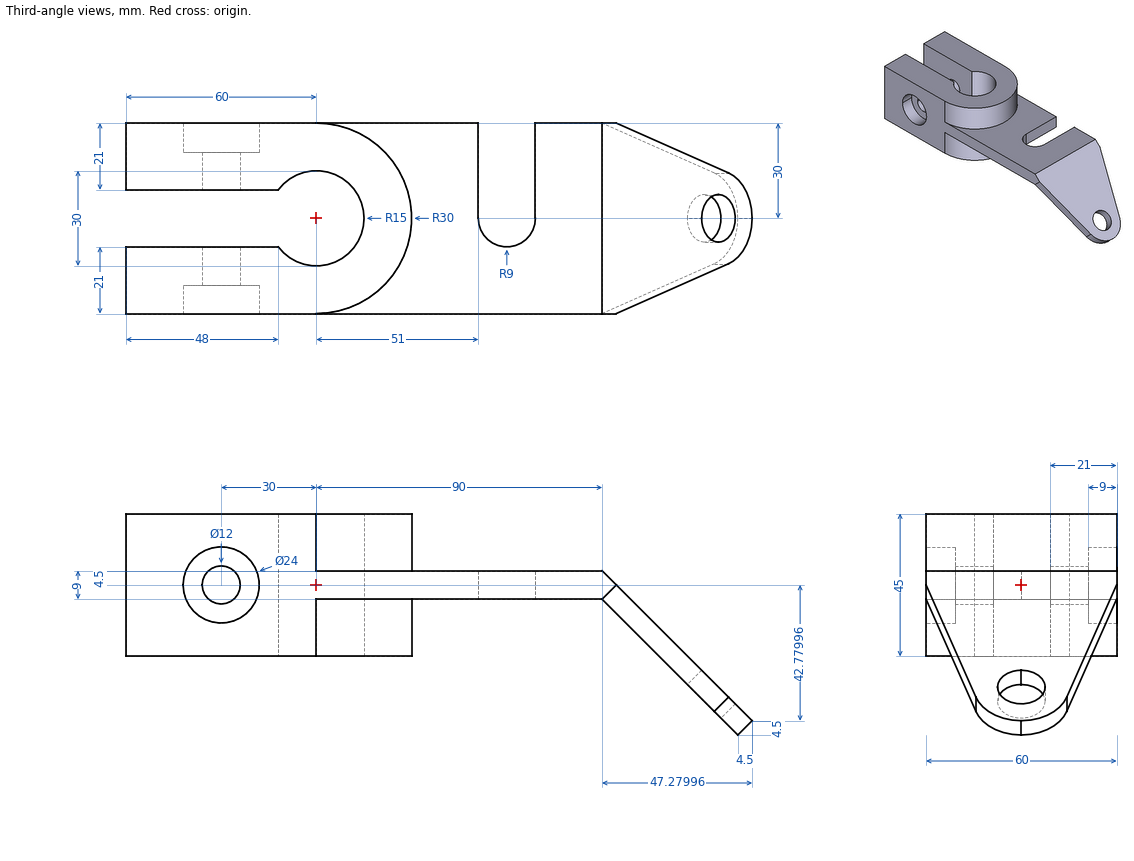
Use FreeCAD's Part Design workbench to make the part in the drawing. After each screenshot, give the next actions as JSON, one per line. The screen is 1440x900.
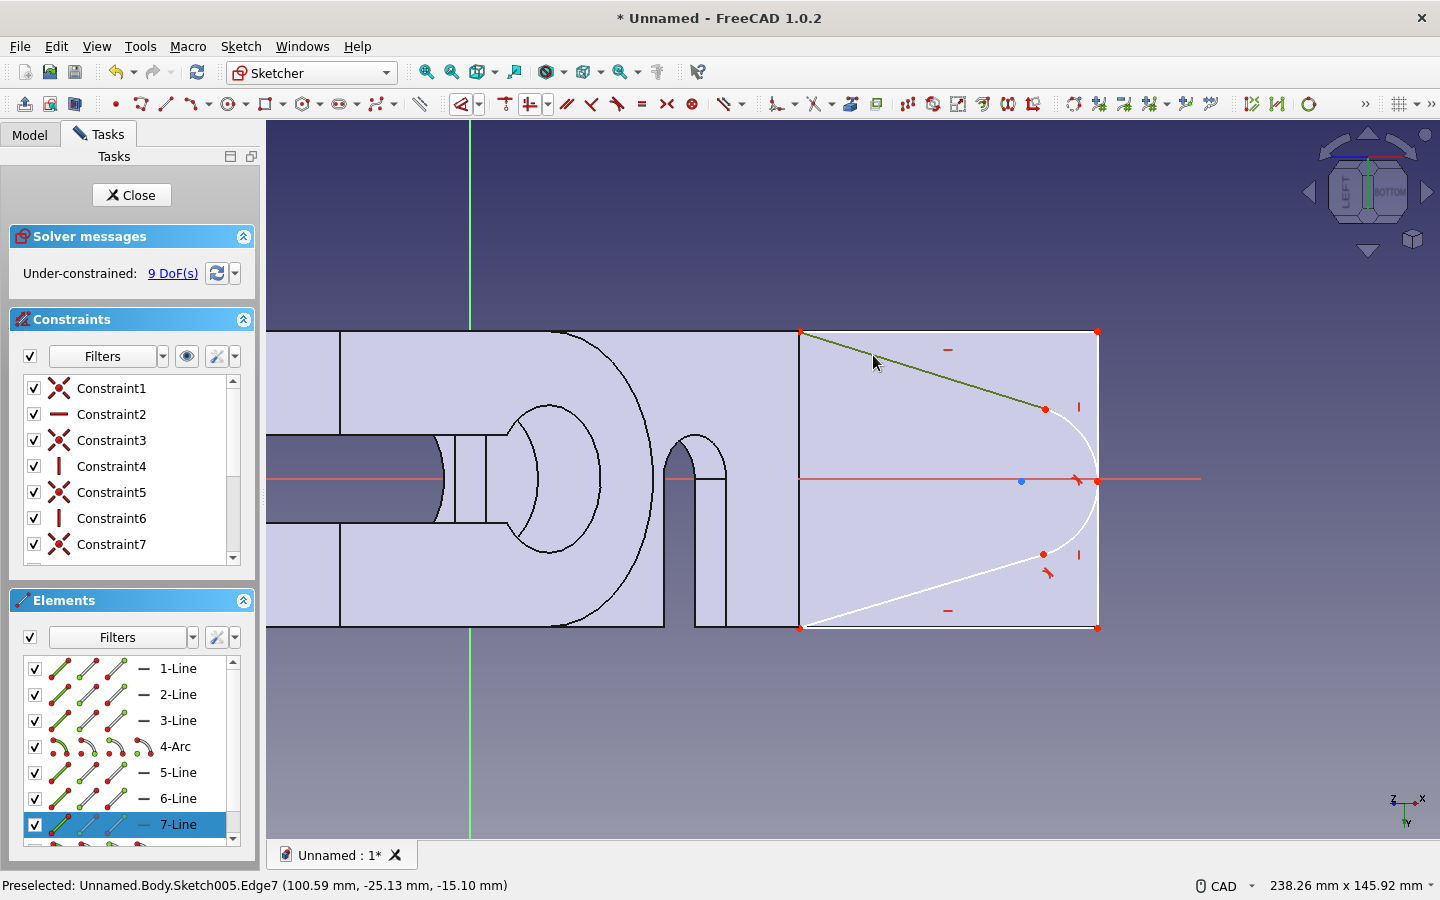
{"action": "left_click", "coordinate": [1071, 423]}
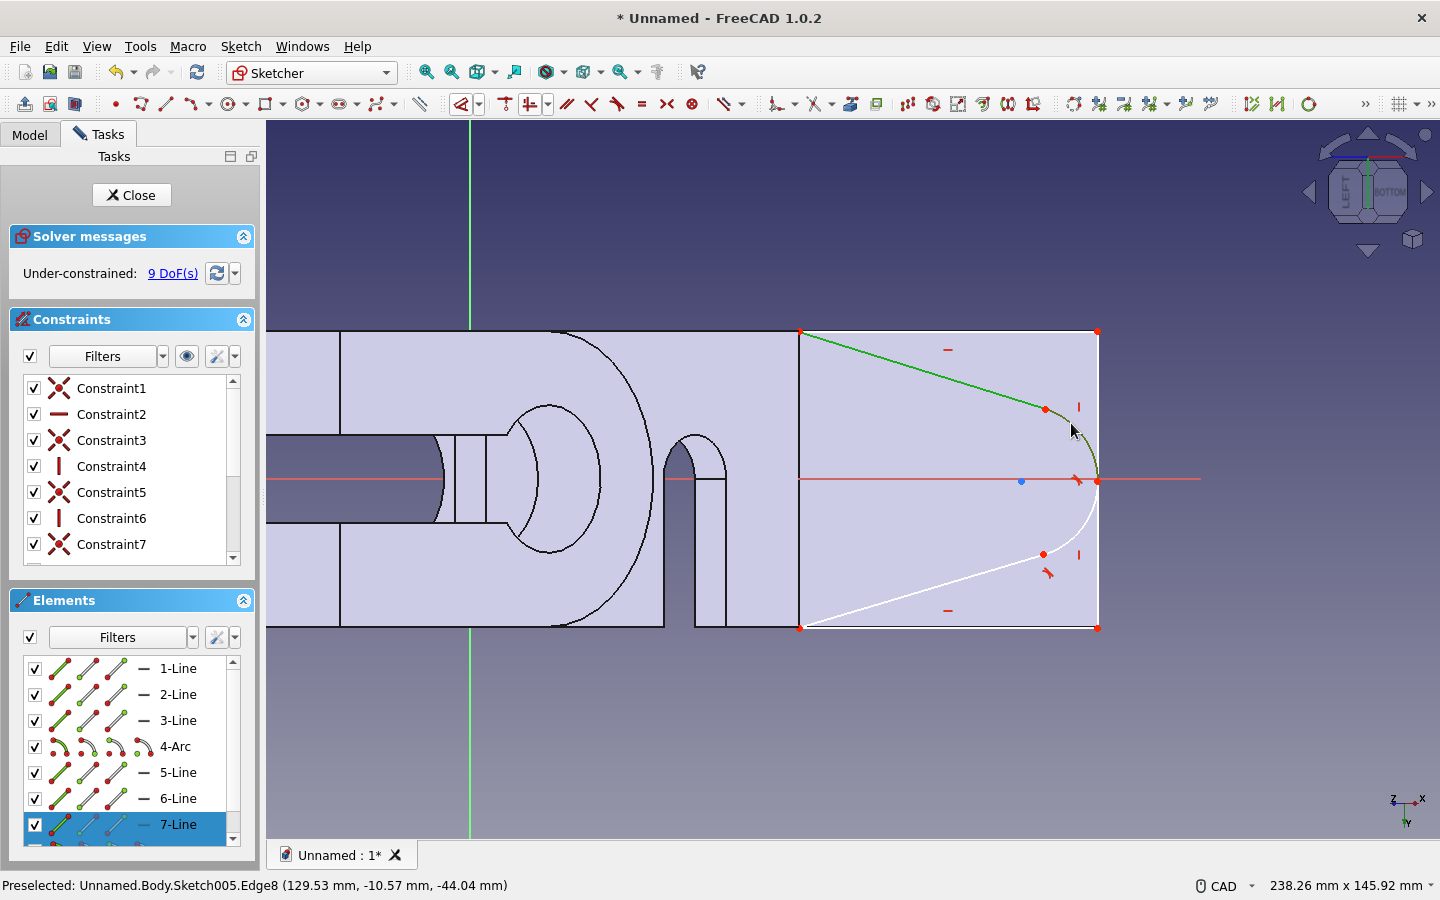
{"action": "left_click", "coordinate": [617, 104]}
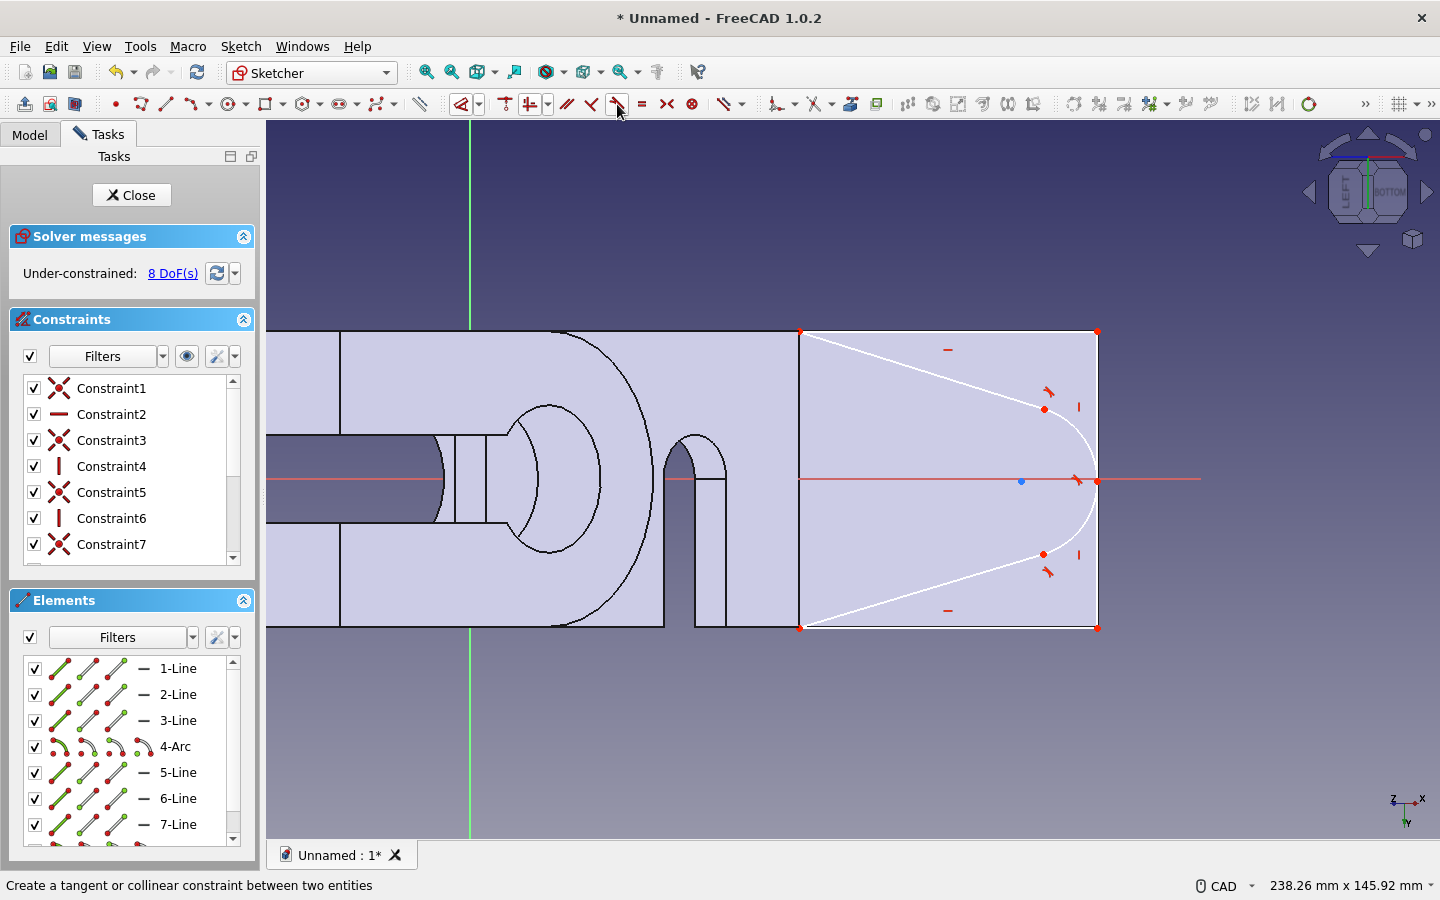
{"action": "left_click", "coordinate": [1069, 541]}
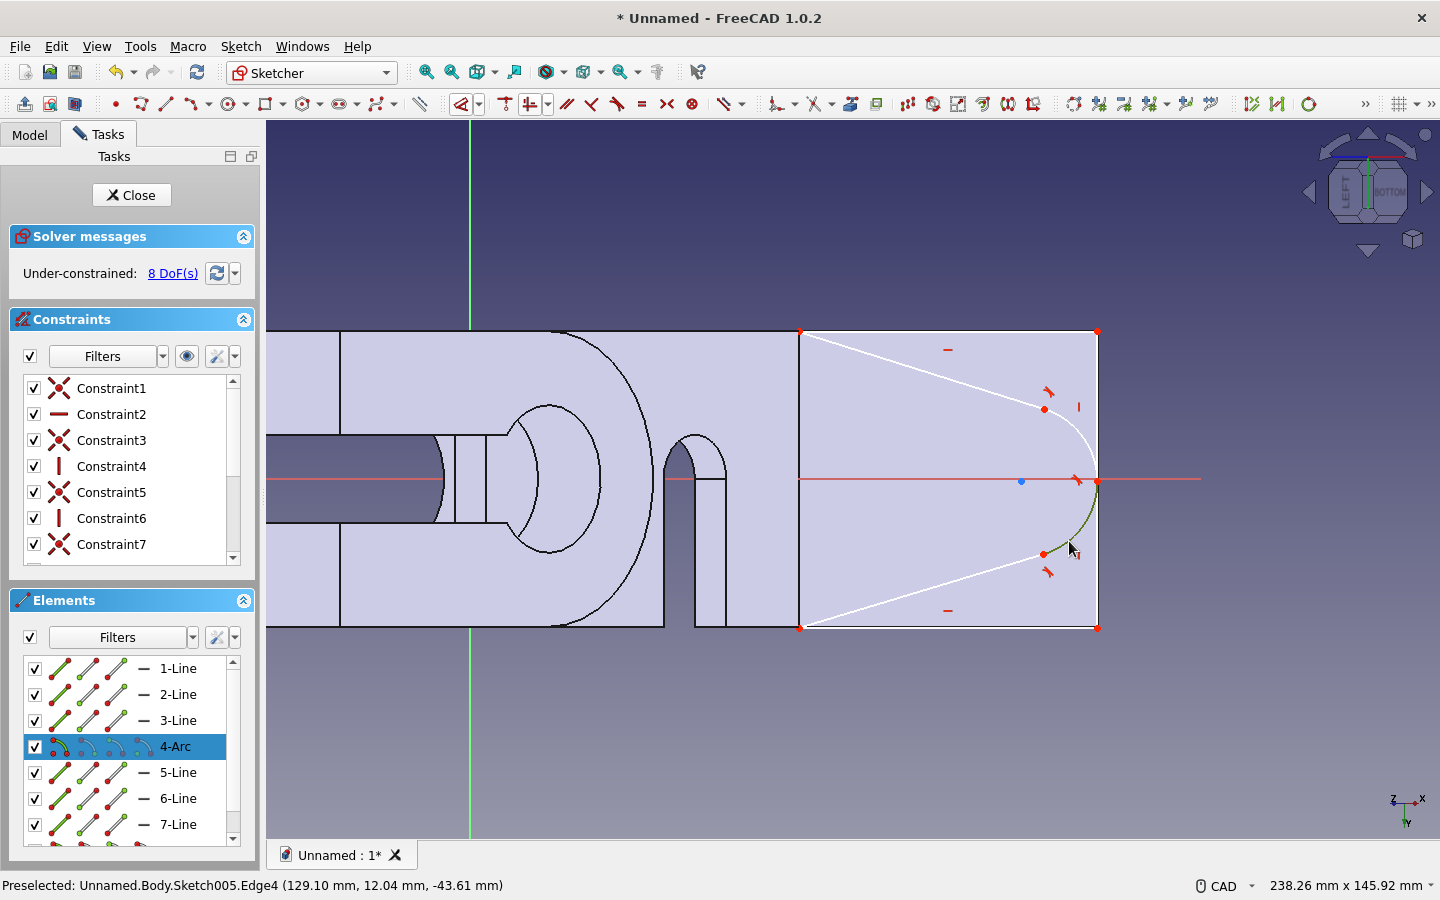
{"action": "left_click", "coordinate": [1069, 423]}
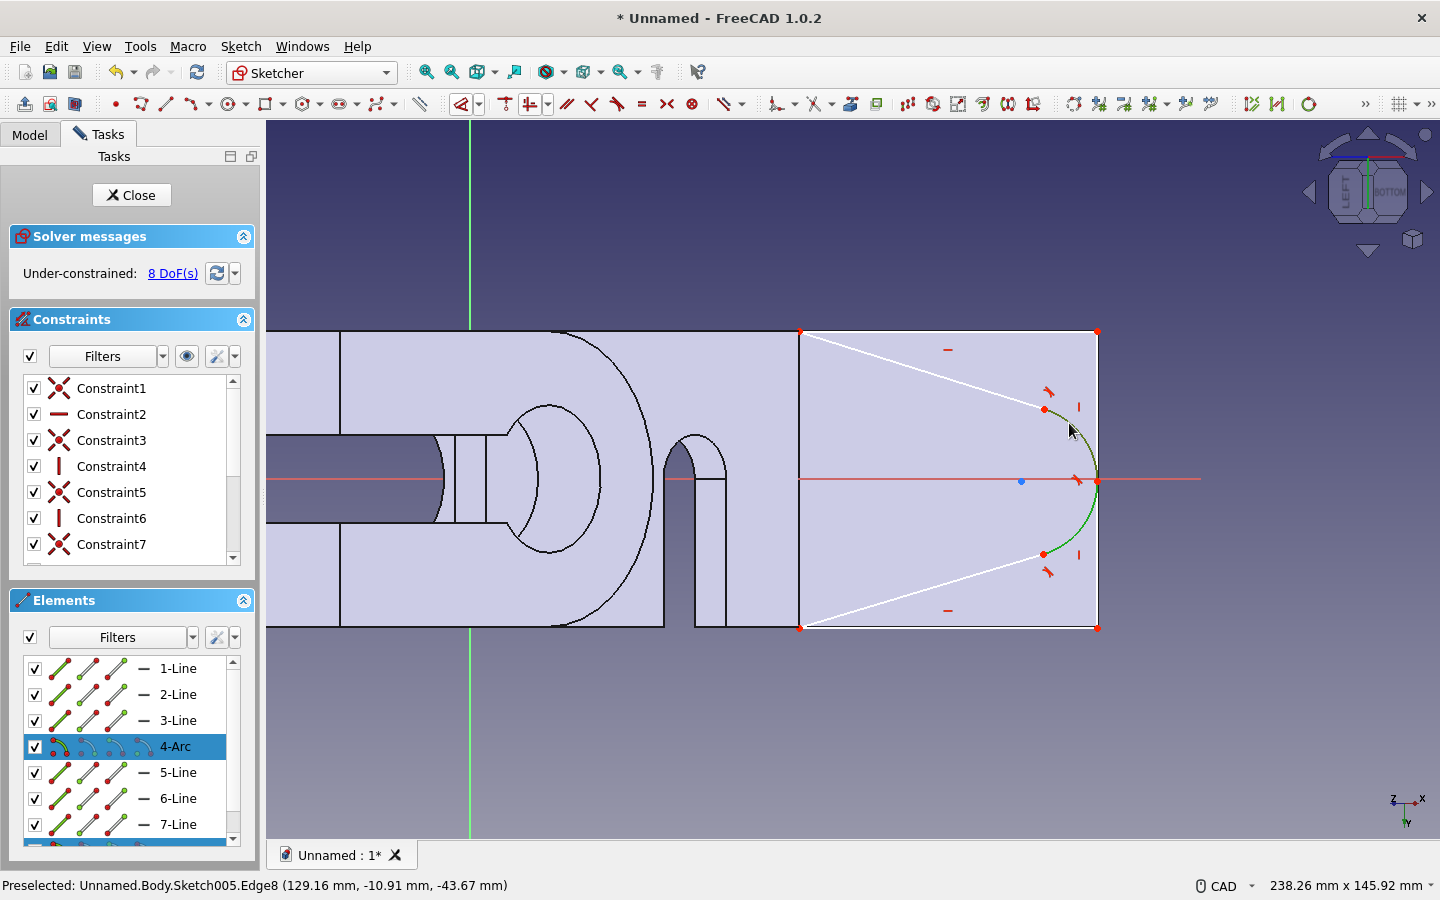
{"action": "left_click", "coordinate": [642, 104]}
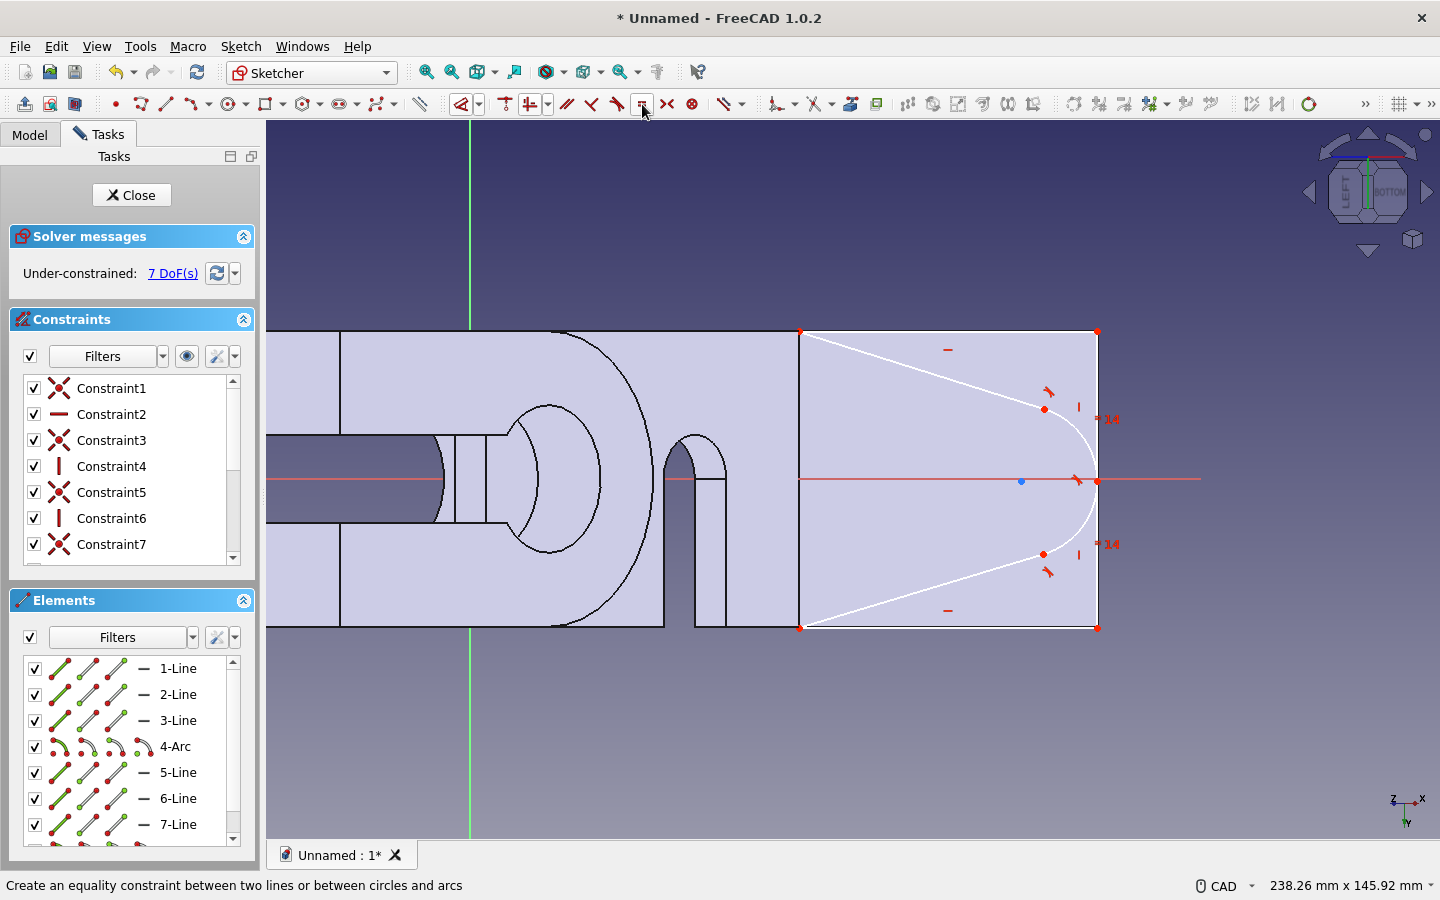
{"action": "left_click", "coordinate": [1021, 482]}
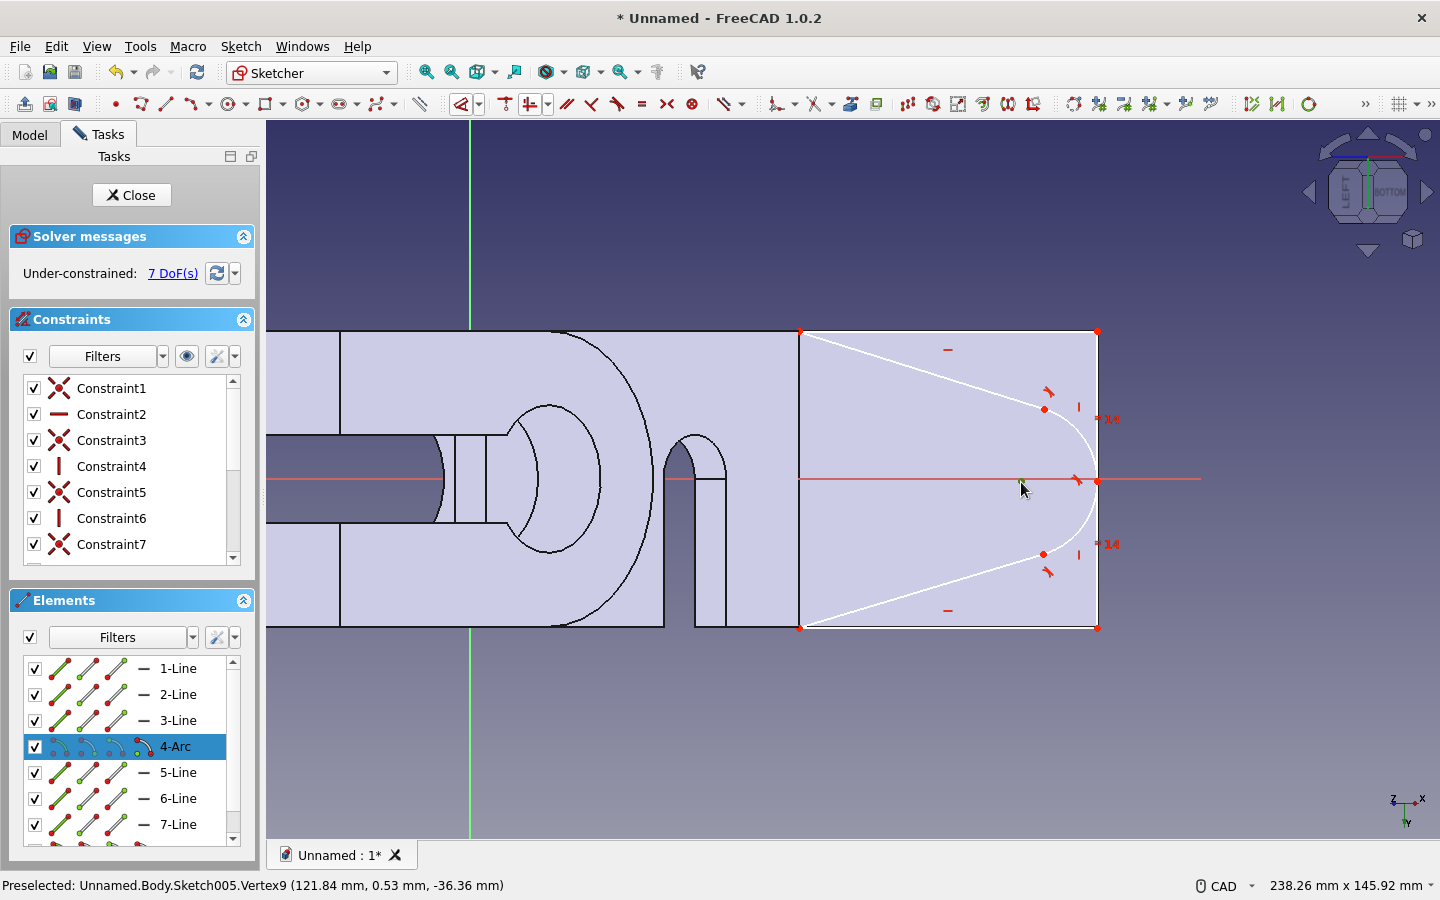
{"action": "left_click", "coordinate": [364, 479]}